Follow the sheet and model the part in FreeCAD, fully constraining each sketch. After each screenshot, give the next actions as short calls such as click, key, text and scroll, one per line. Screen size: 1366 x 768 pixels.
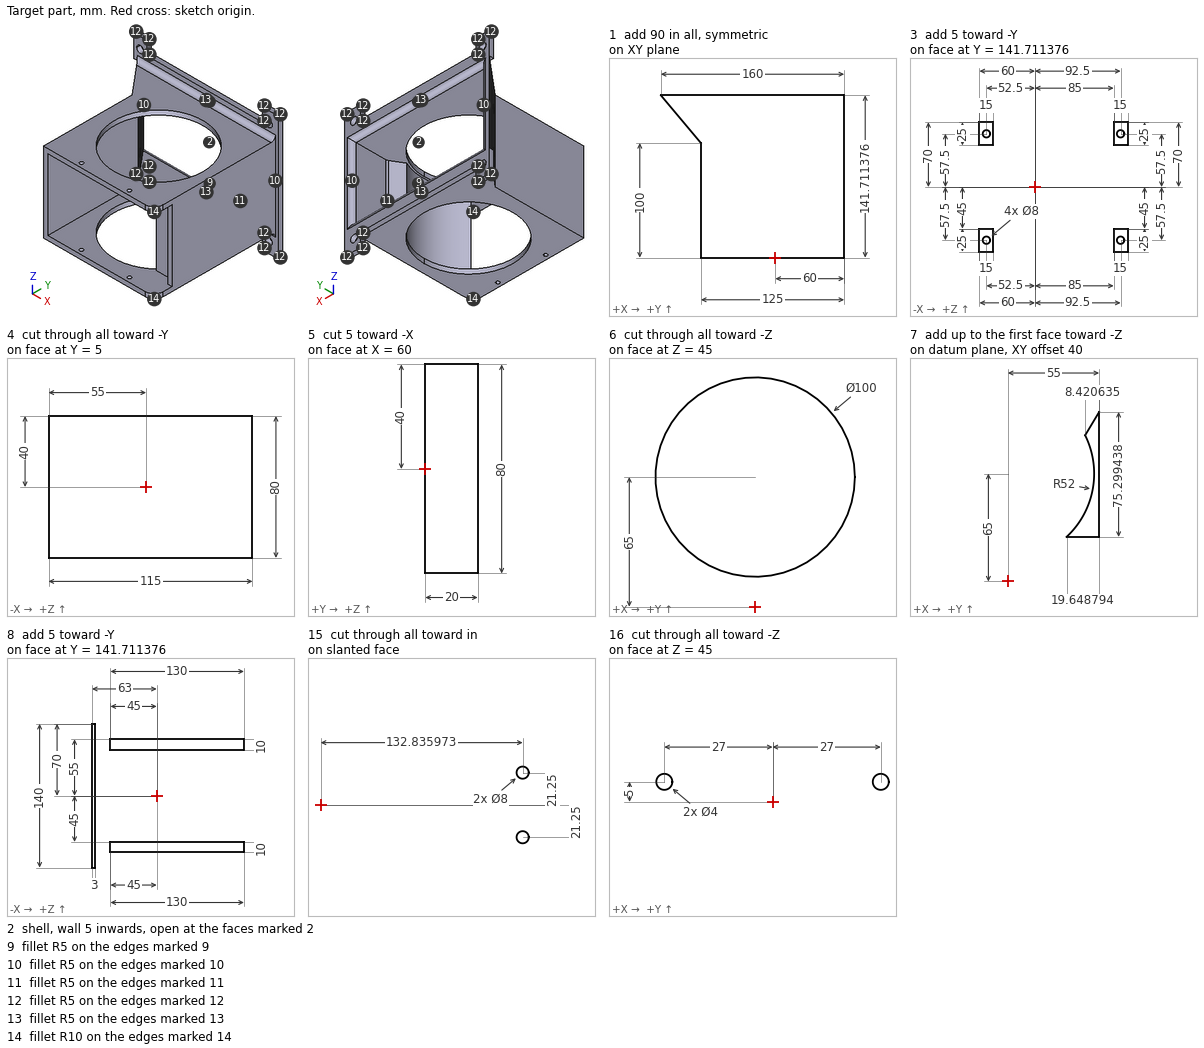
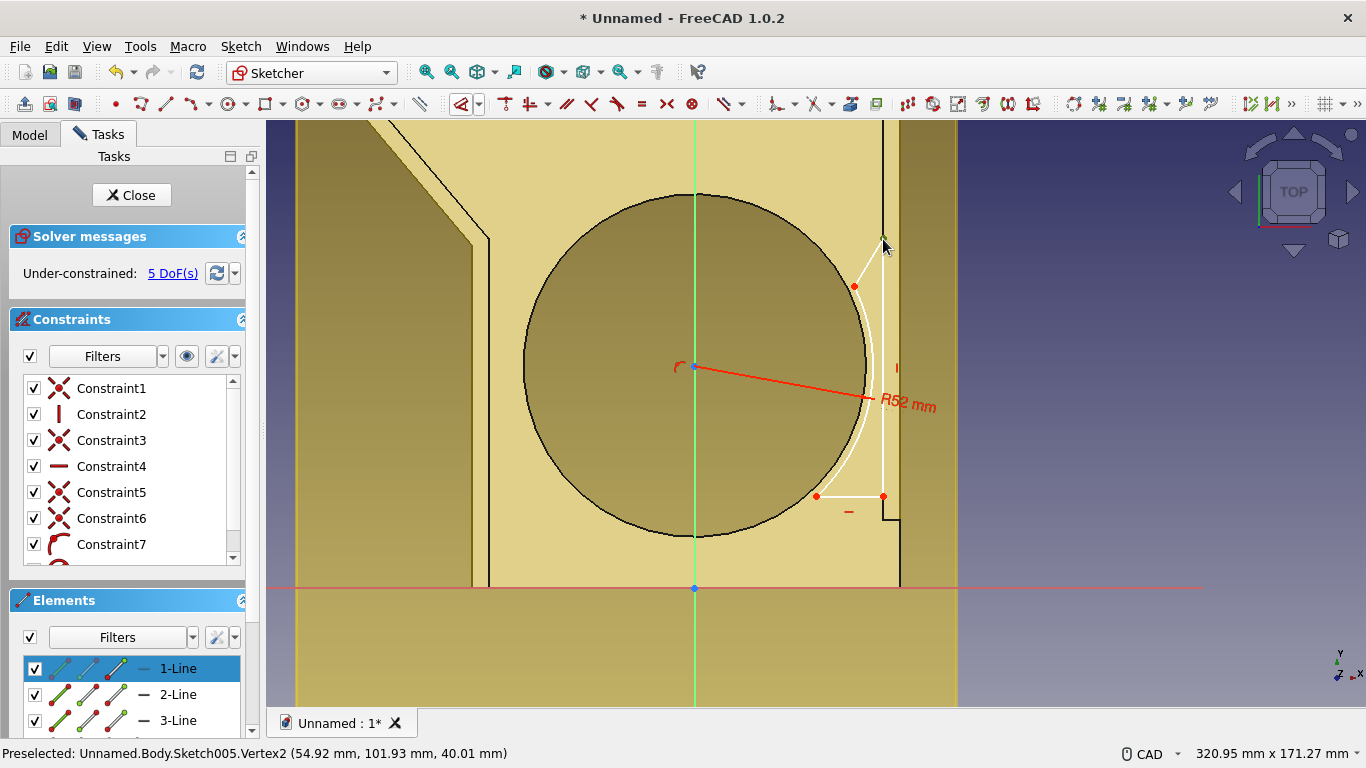
key(l)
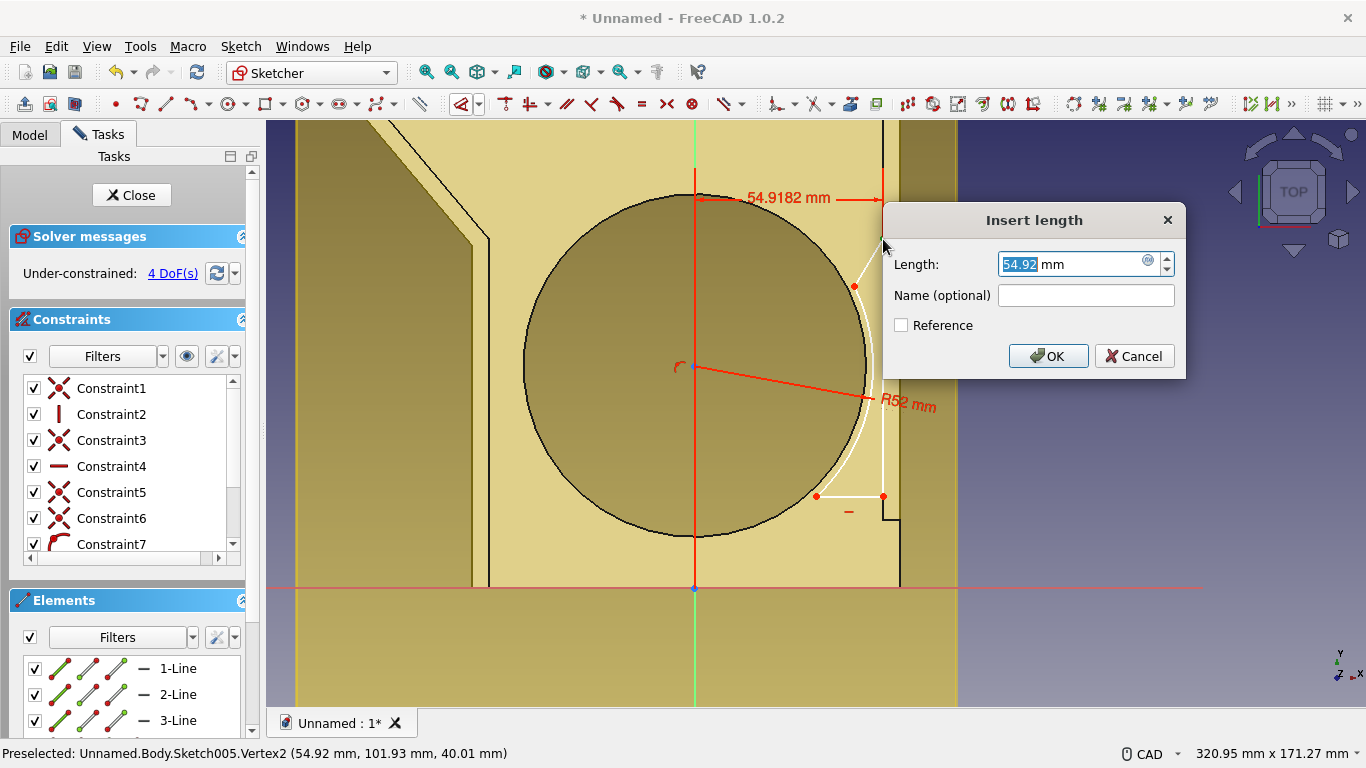
text(55)
key(Return)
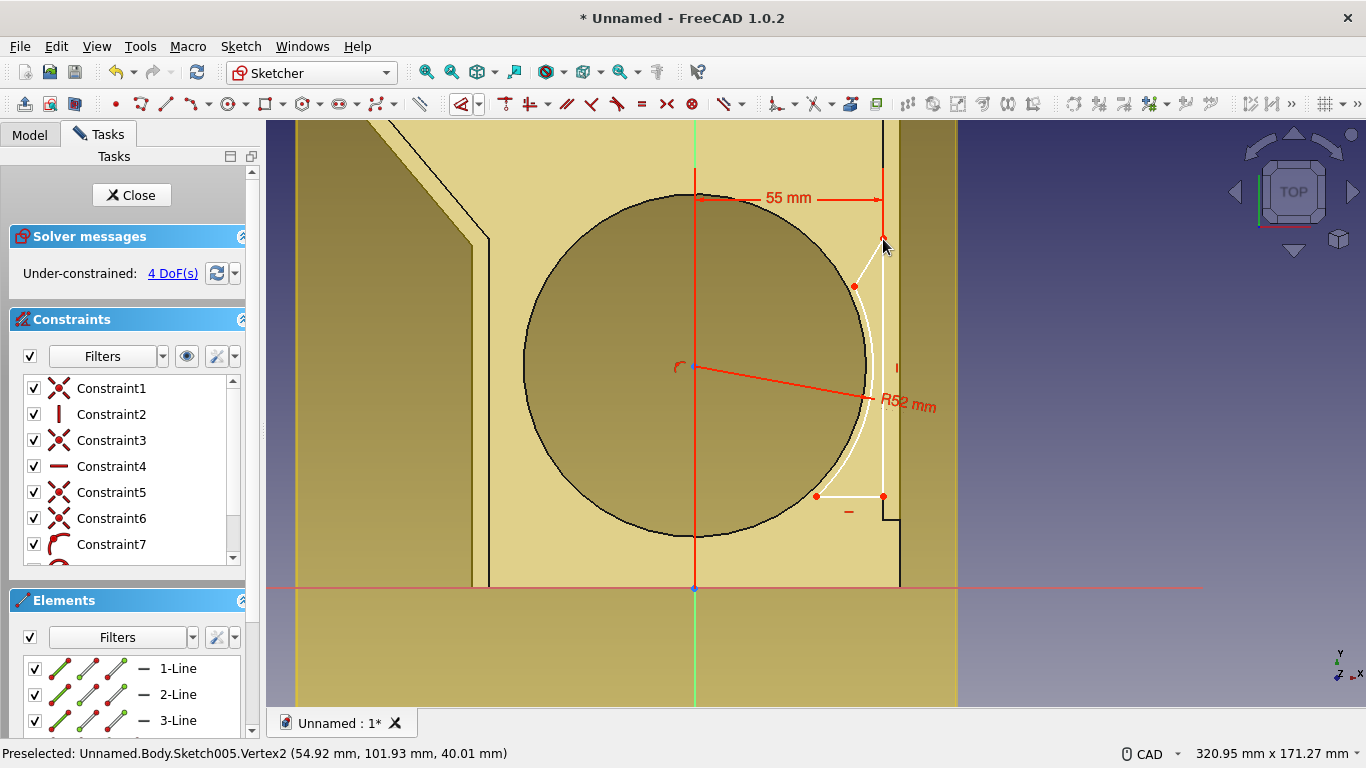
click(695, 366)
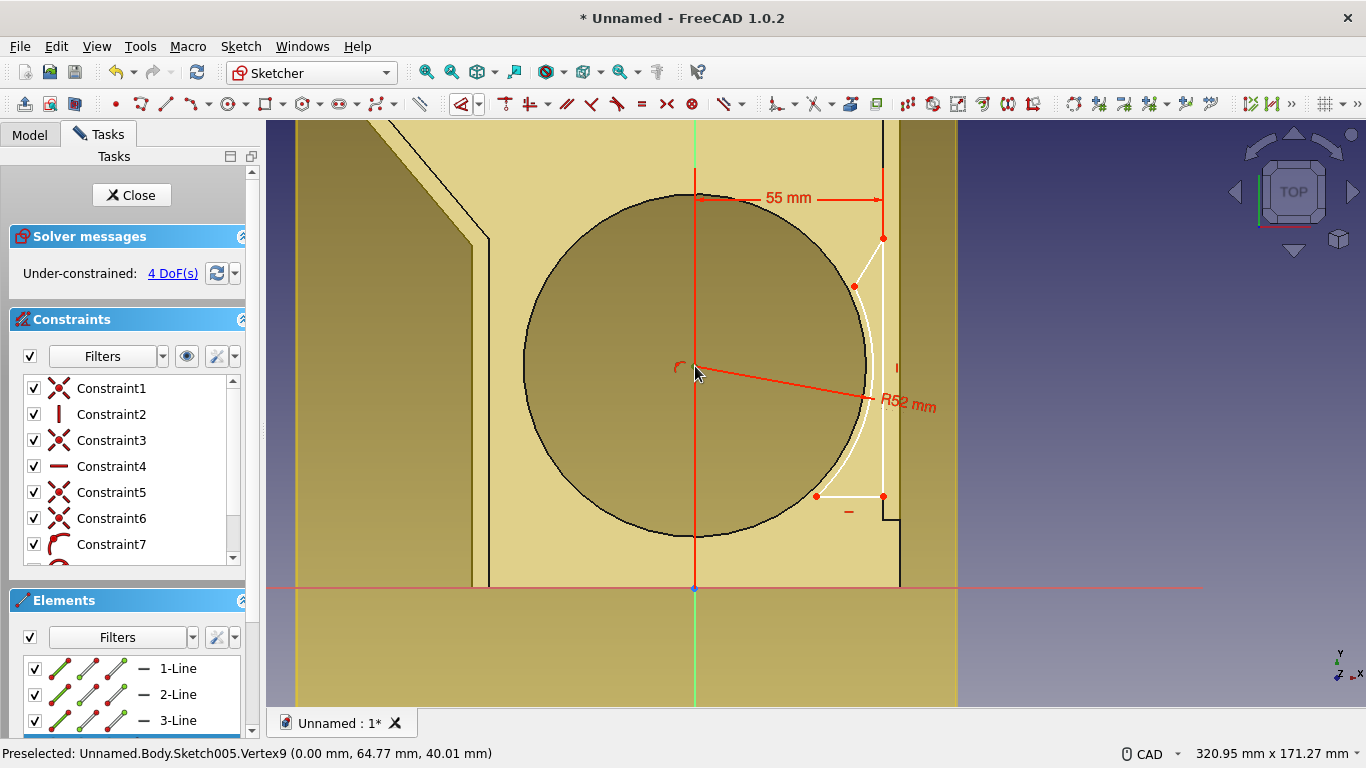
key(i)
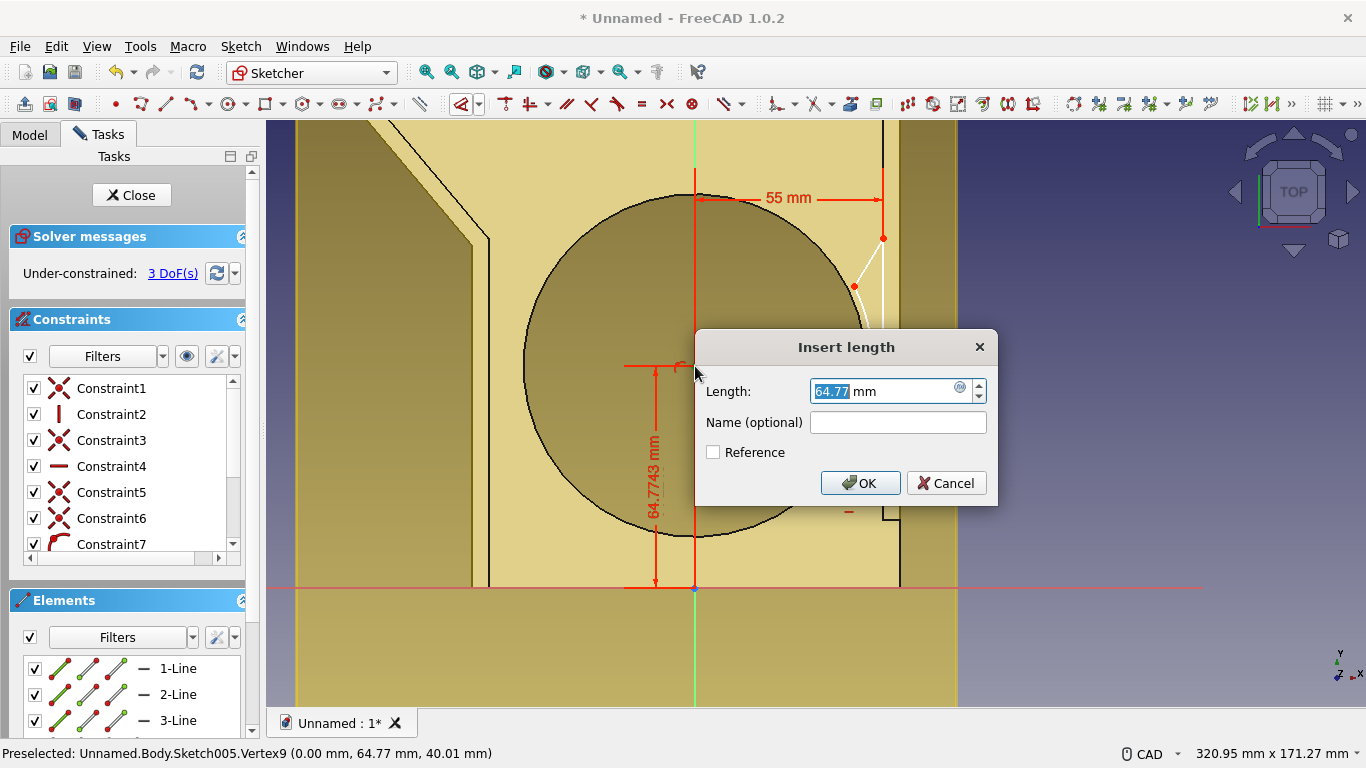
text(65)
key(Return)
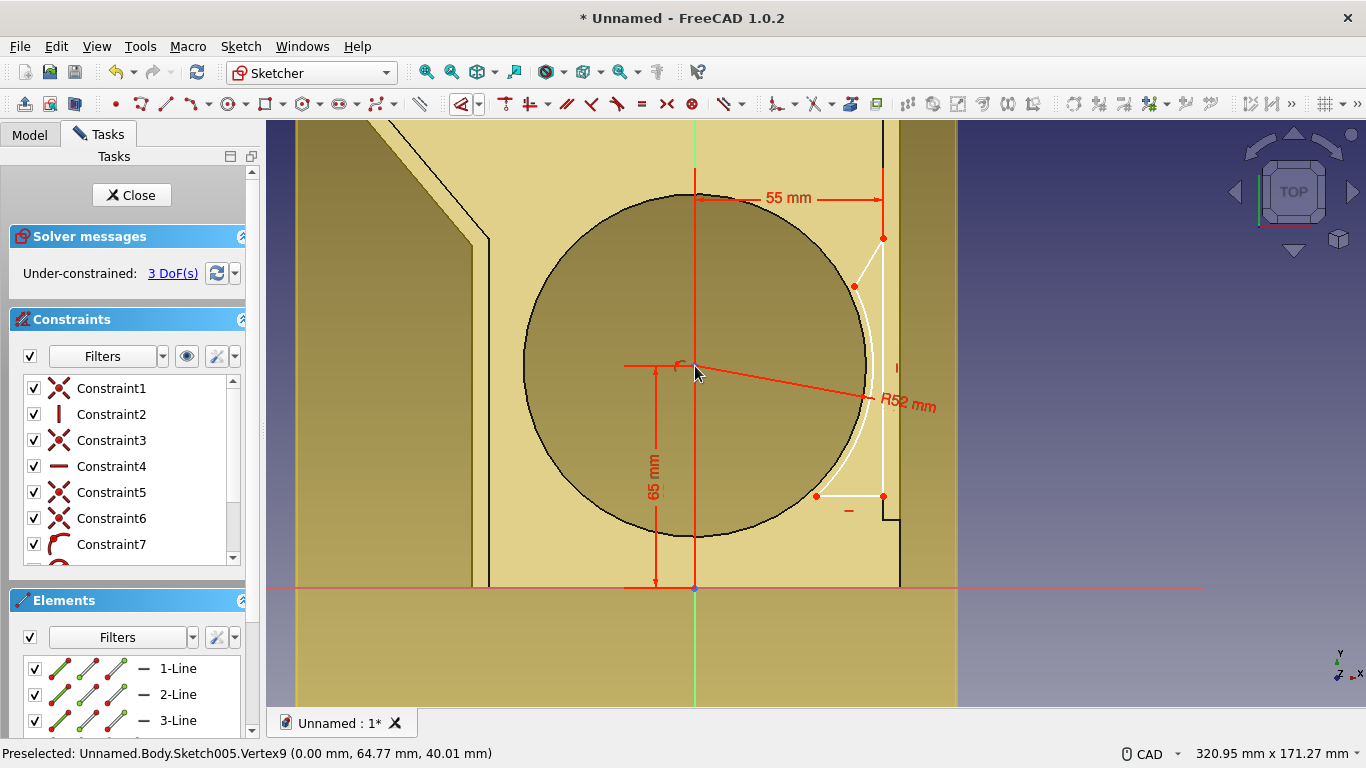
click(883, 316)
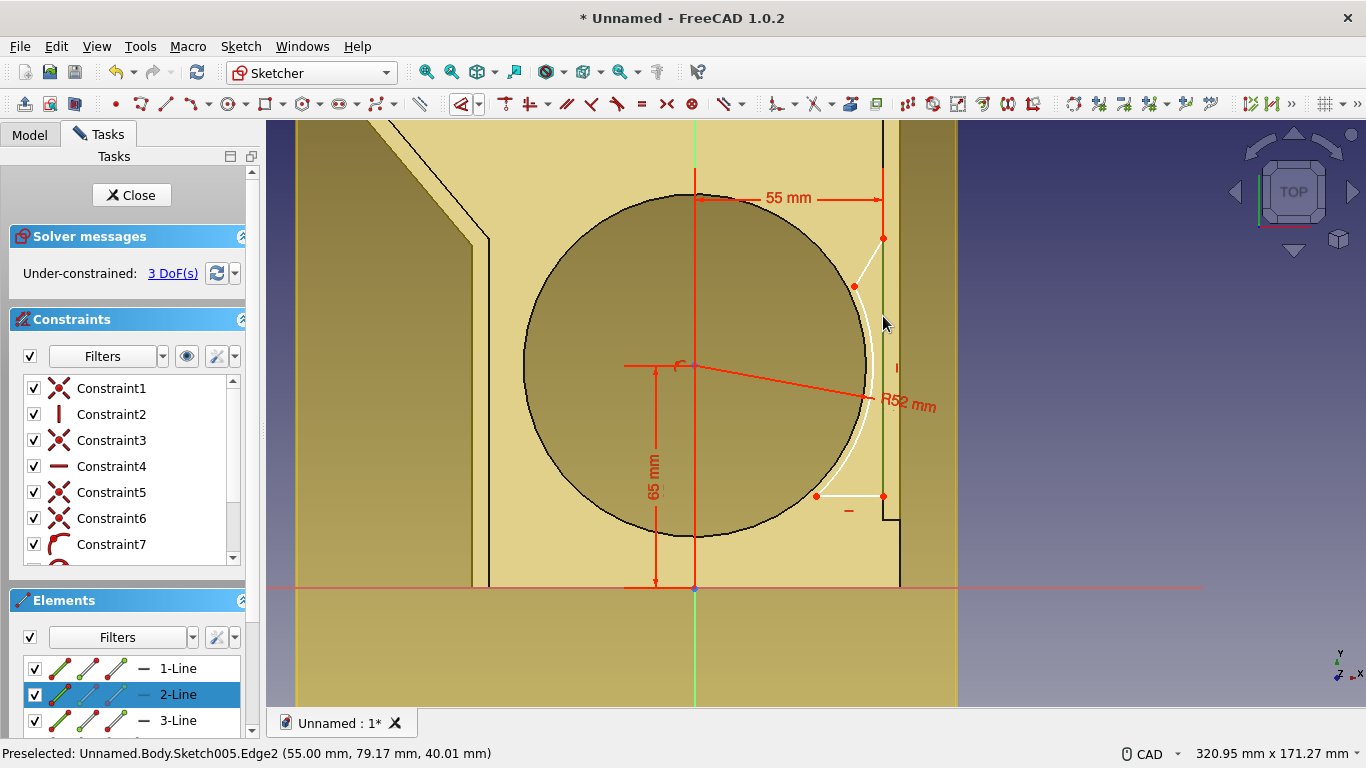
key(i)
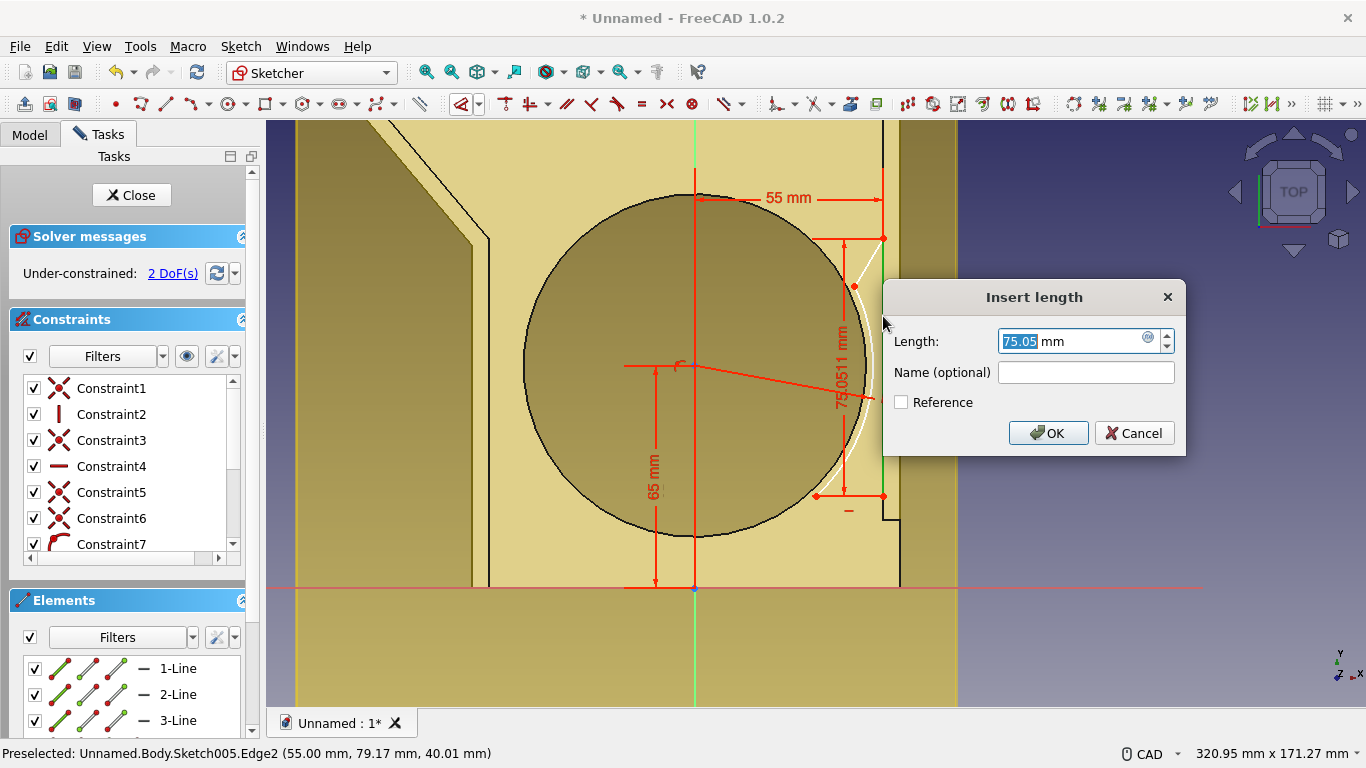
text(75.299438)
key(Return)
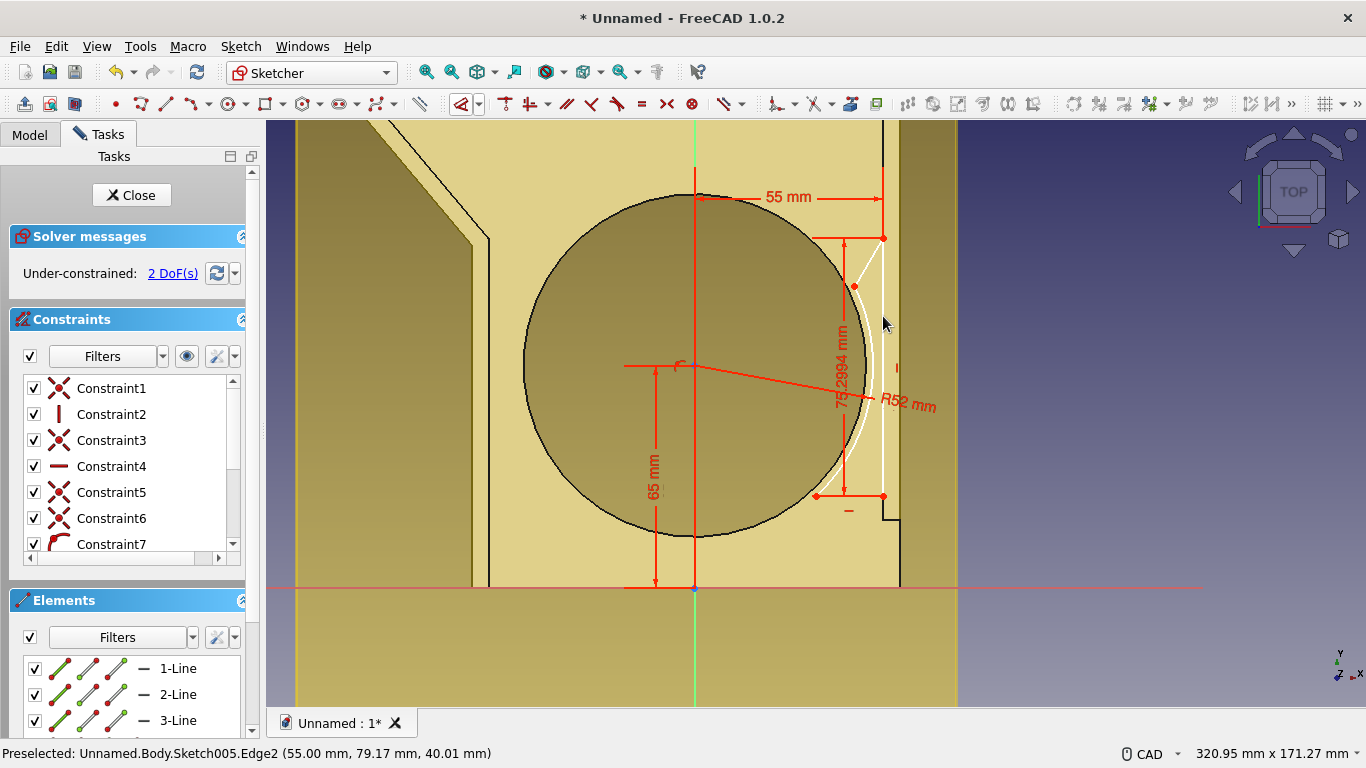
click(863, 496)